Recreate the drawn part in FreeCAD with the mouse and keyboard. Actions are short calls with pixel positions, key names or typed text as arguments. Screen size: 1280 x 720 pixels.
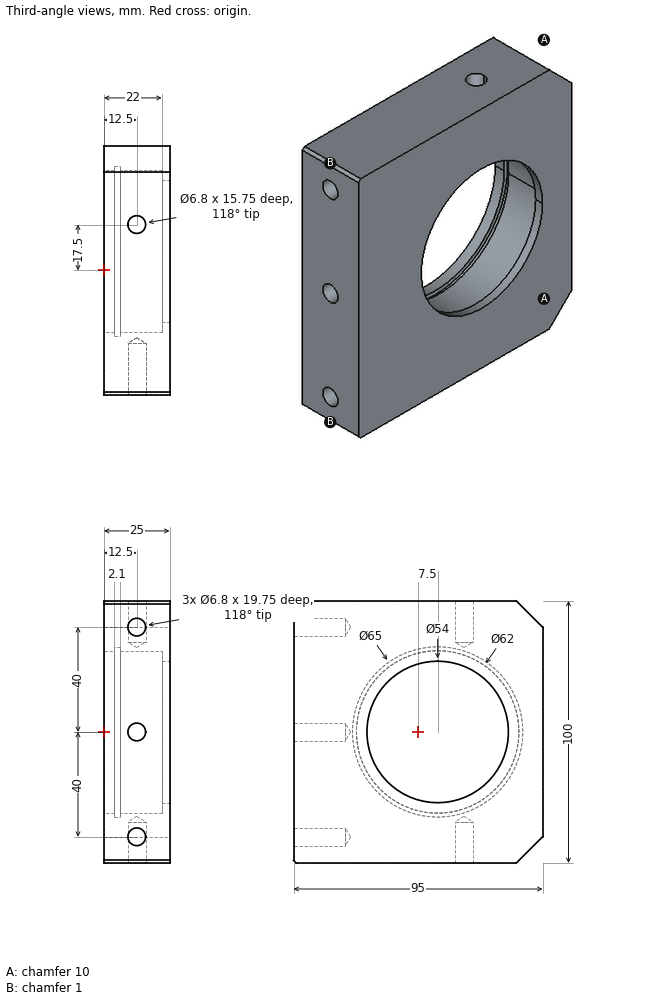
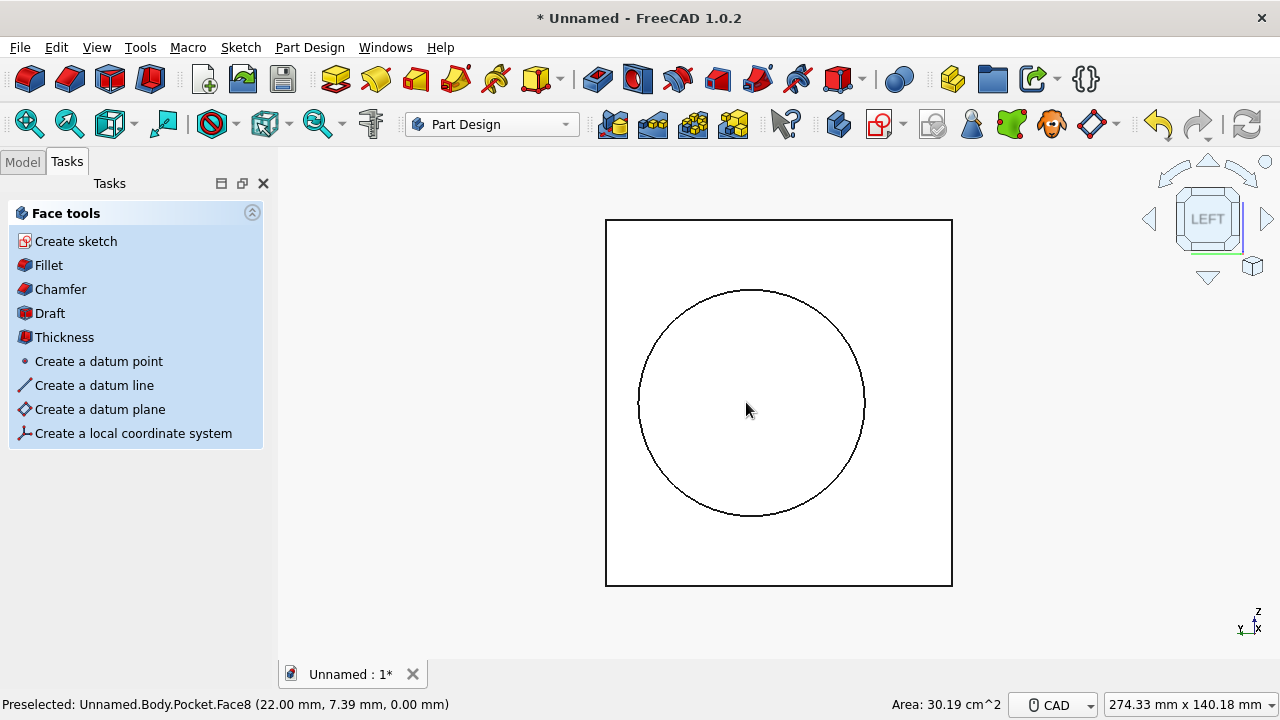
click(880, 124)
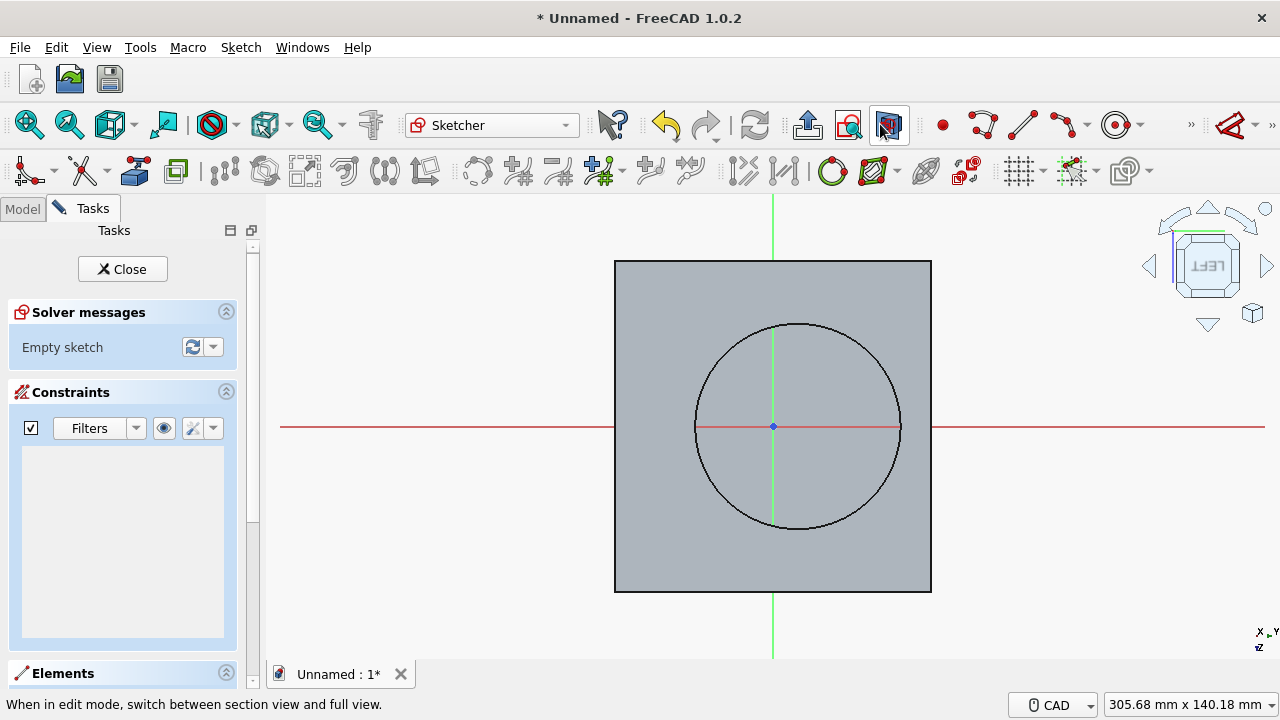
scroll(988, 426, up, 2)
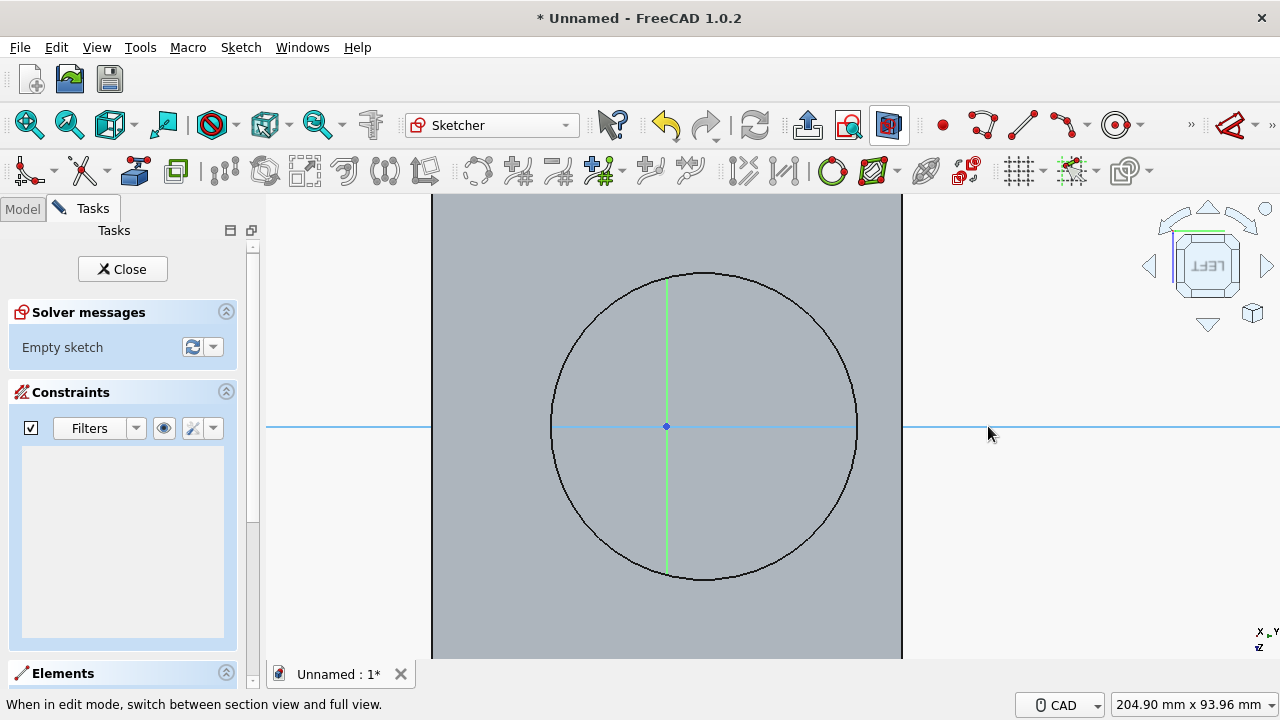
click(1116, 126)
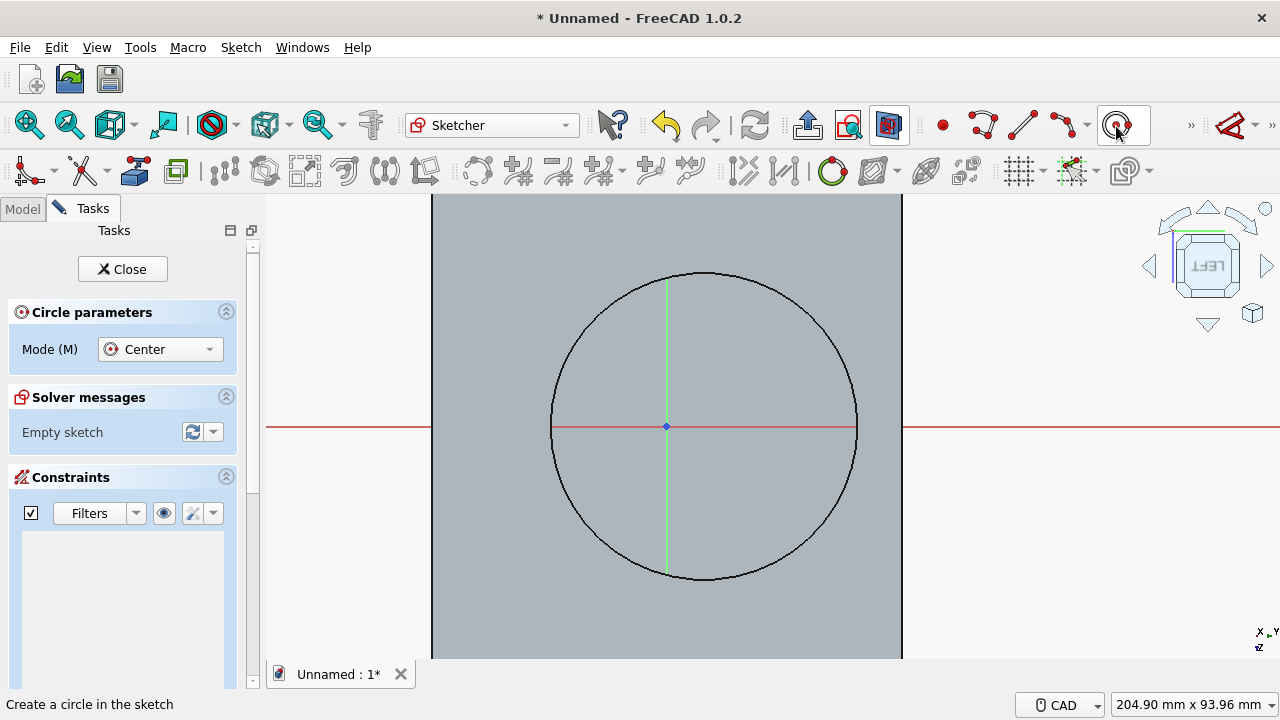
click(704, 426)
click(799, 332)
key(Escape)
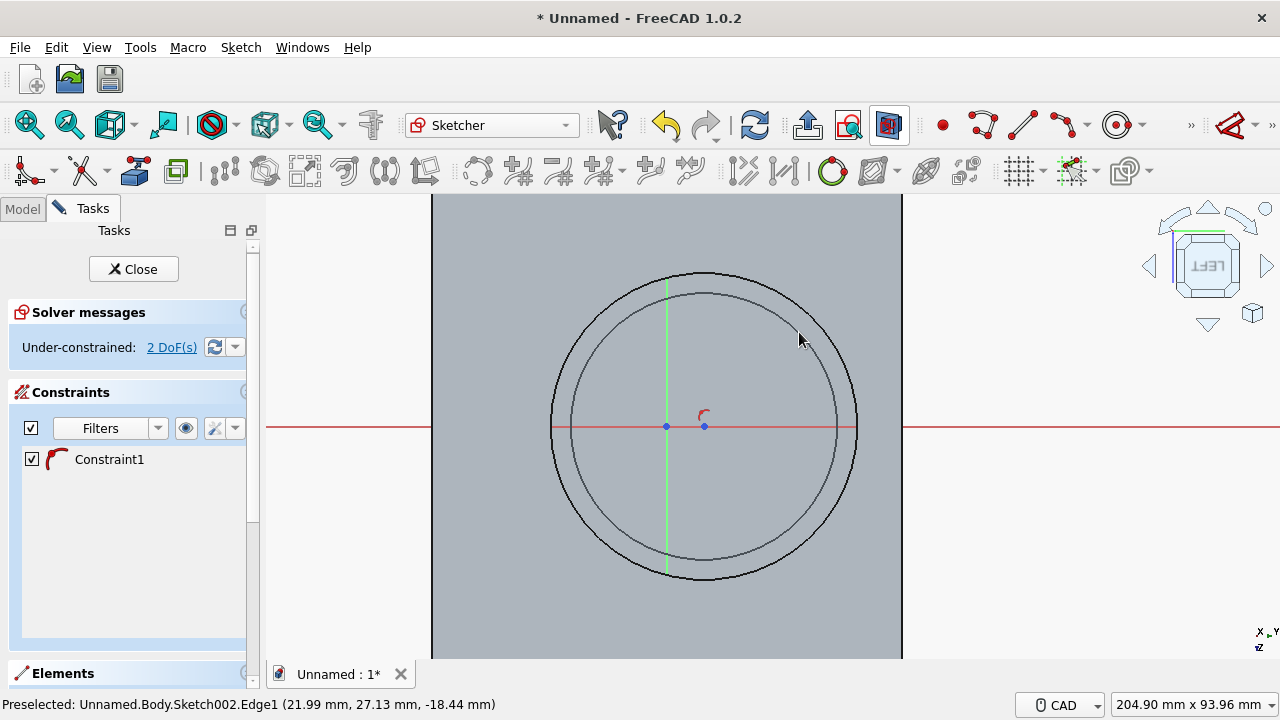
click(1230, 126)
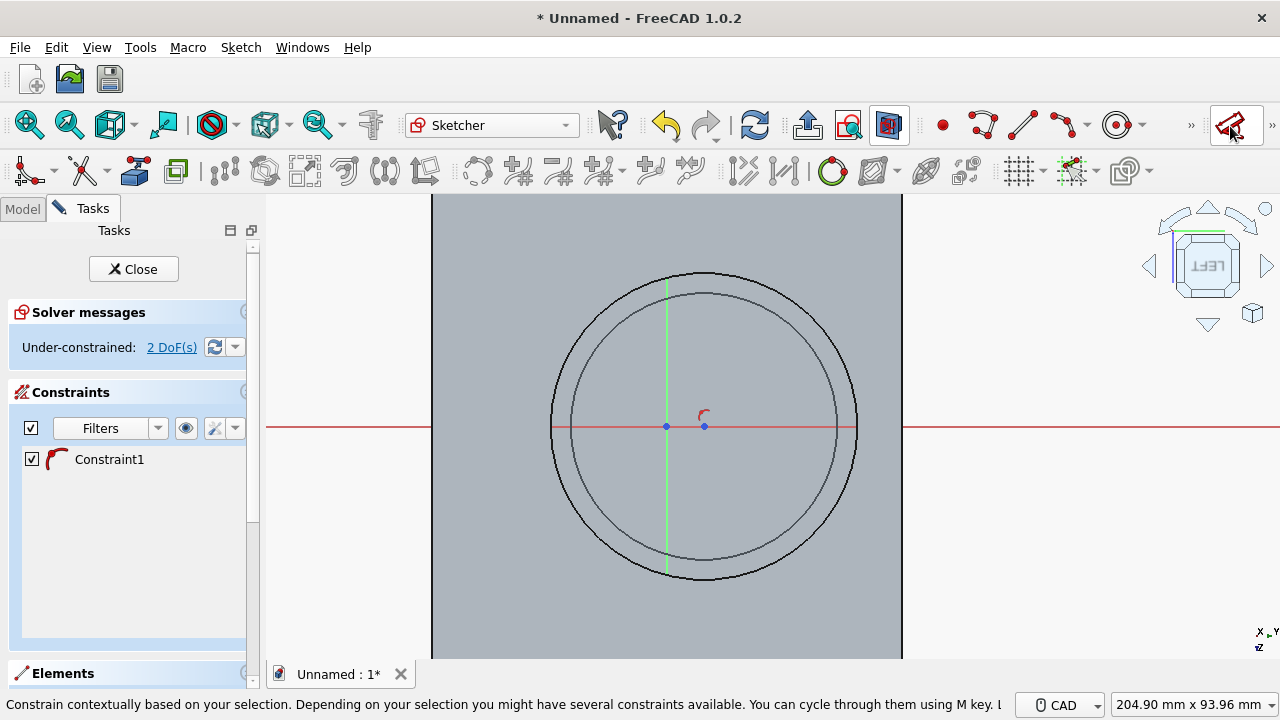
click(798, 332)
click(821, 309)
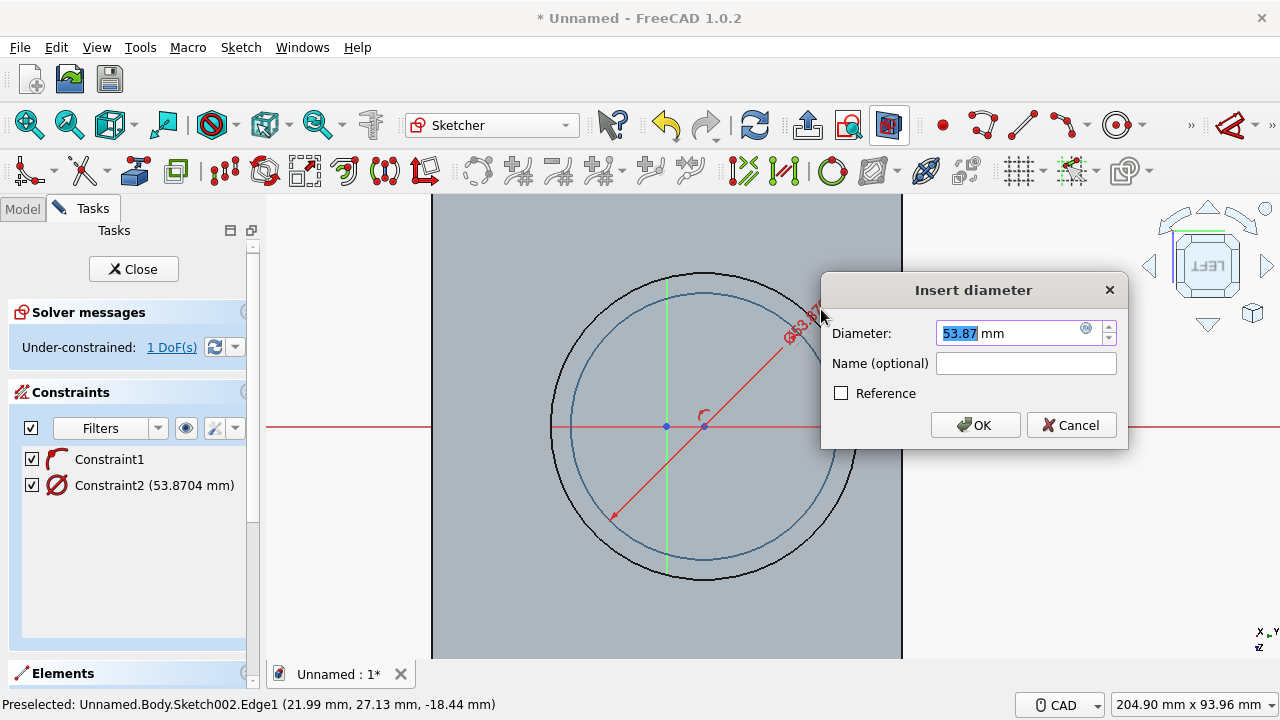
text(54)
key(Return)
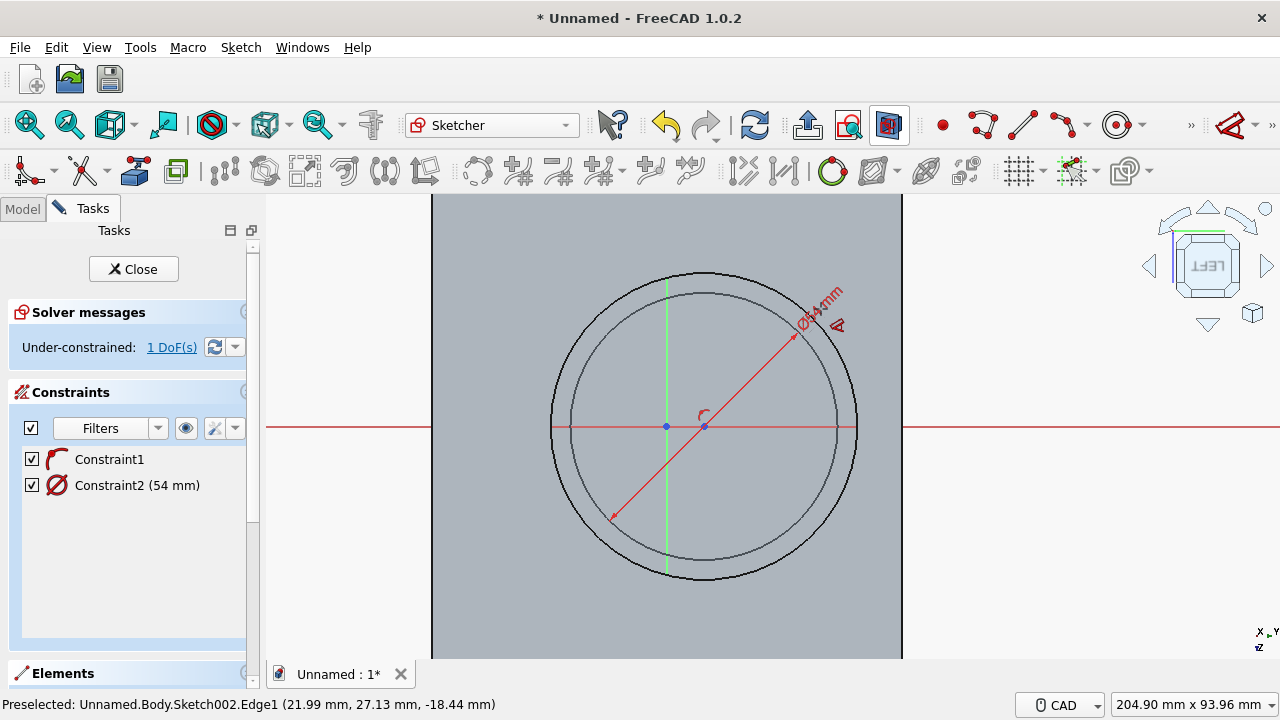
click(704, 426)
click(685, 460)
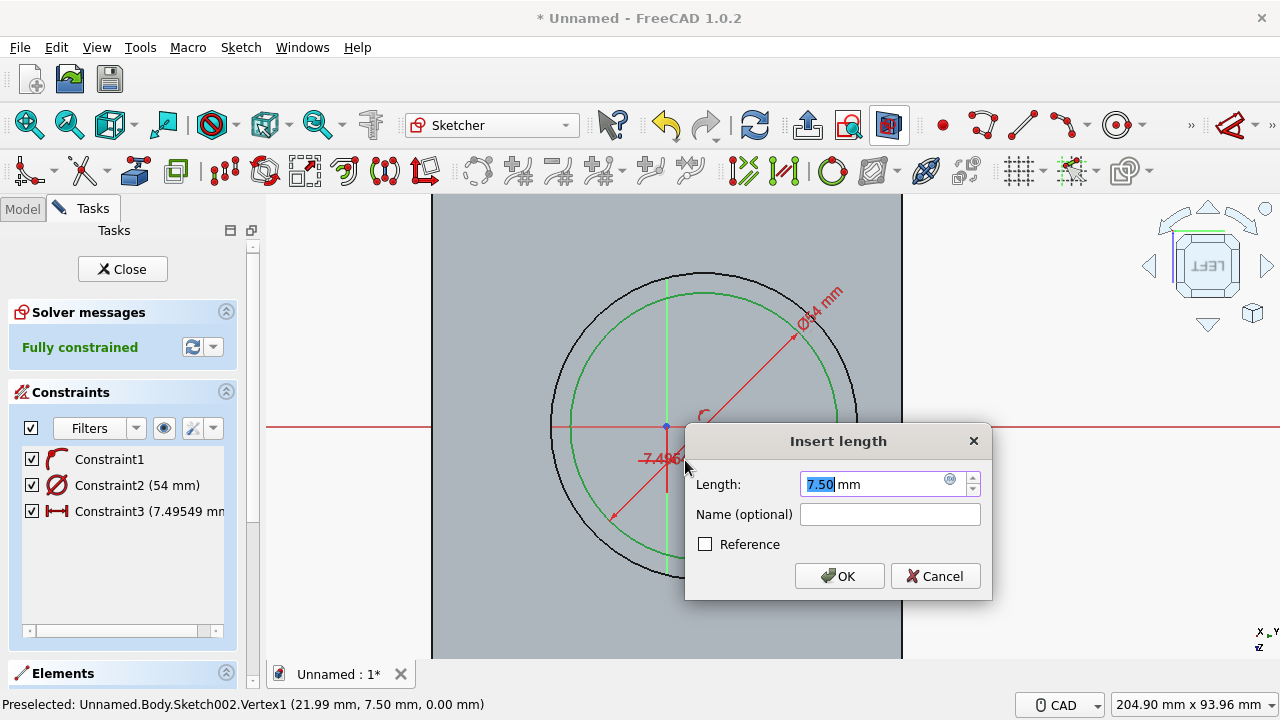
text(7.5)
key(Return)
key(Escape)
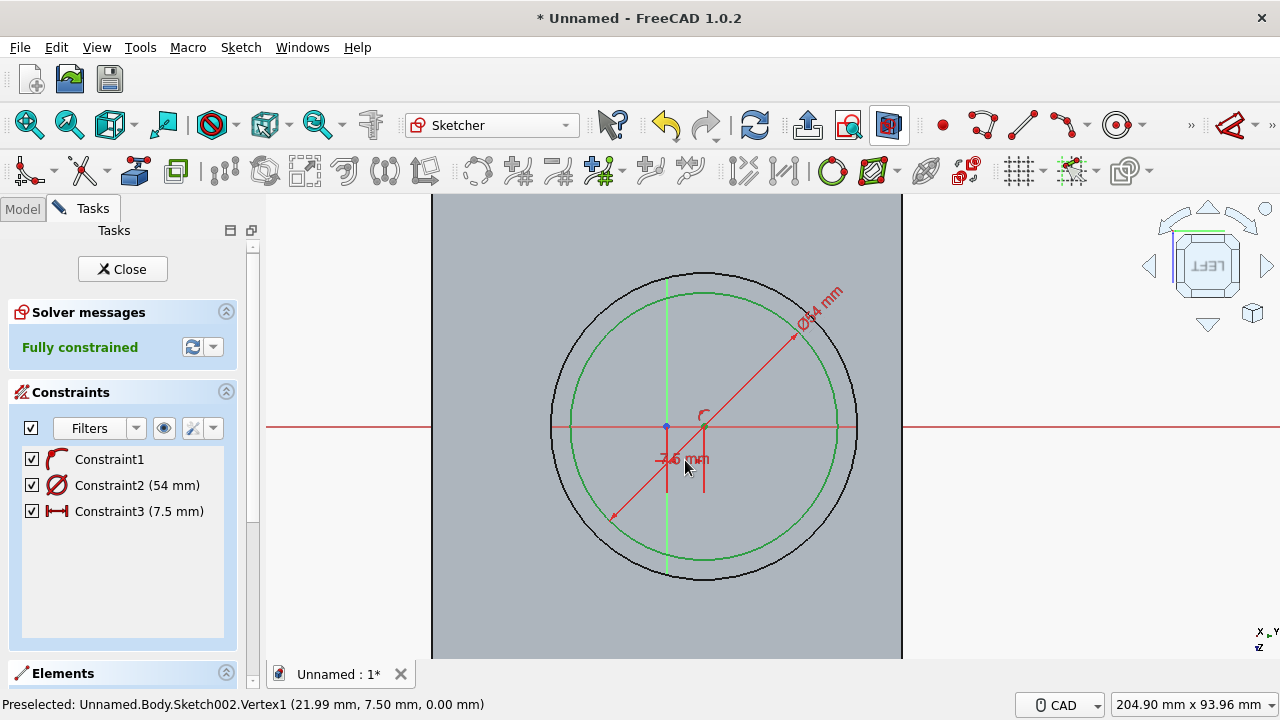
click(123, 269)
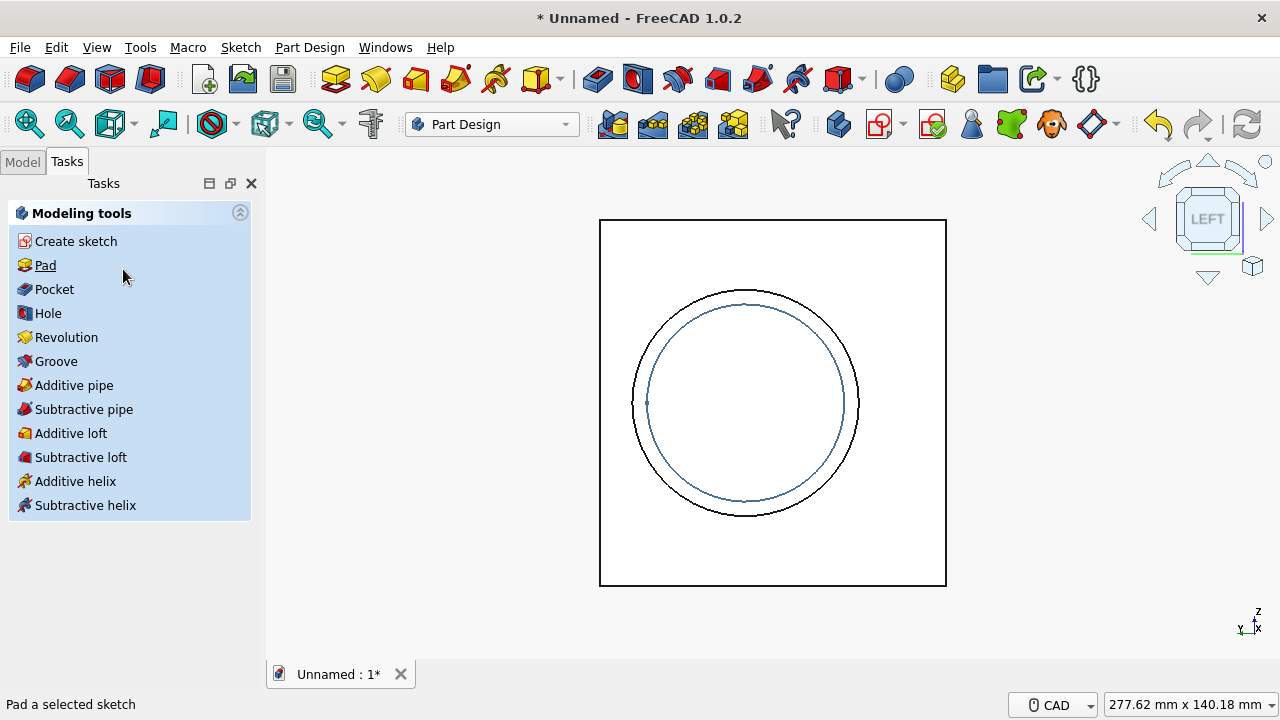
click(598, 80)